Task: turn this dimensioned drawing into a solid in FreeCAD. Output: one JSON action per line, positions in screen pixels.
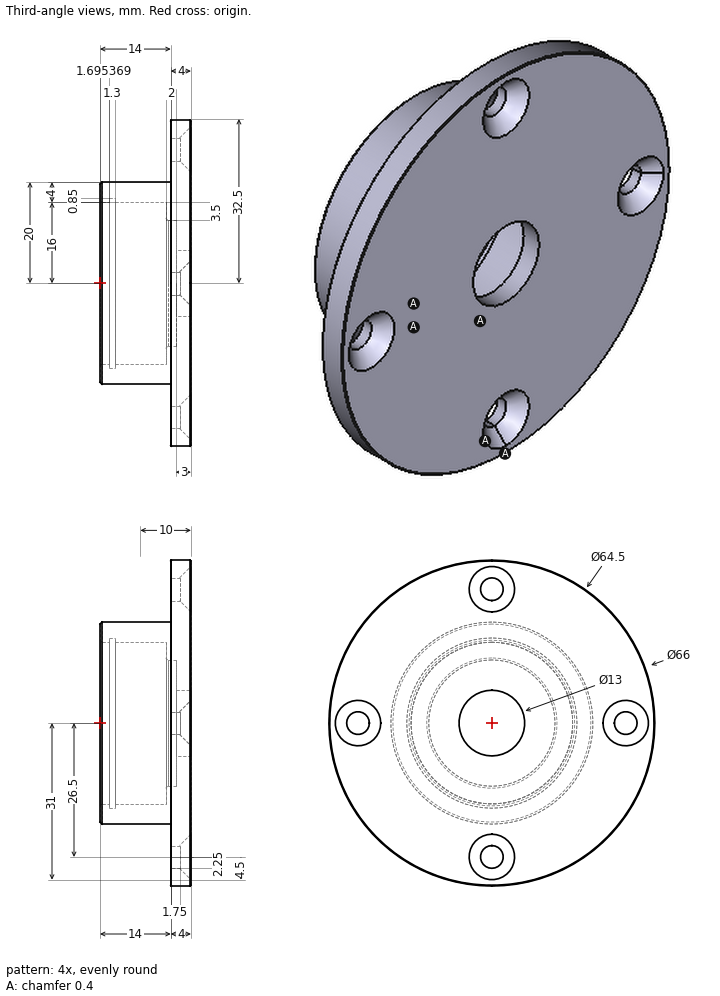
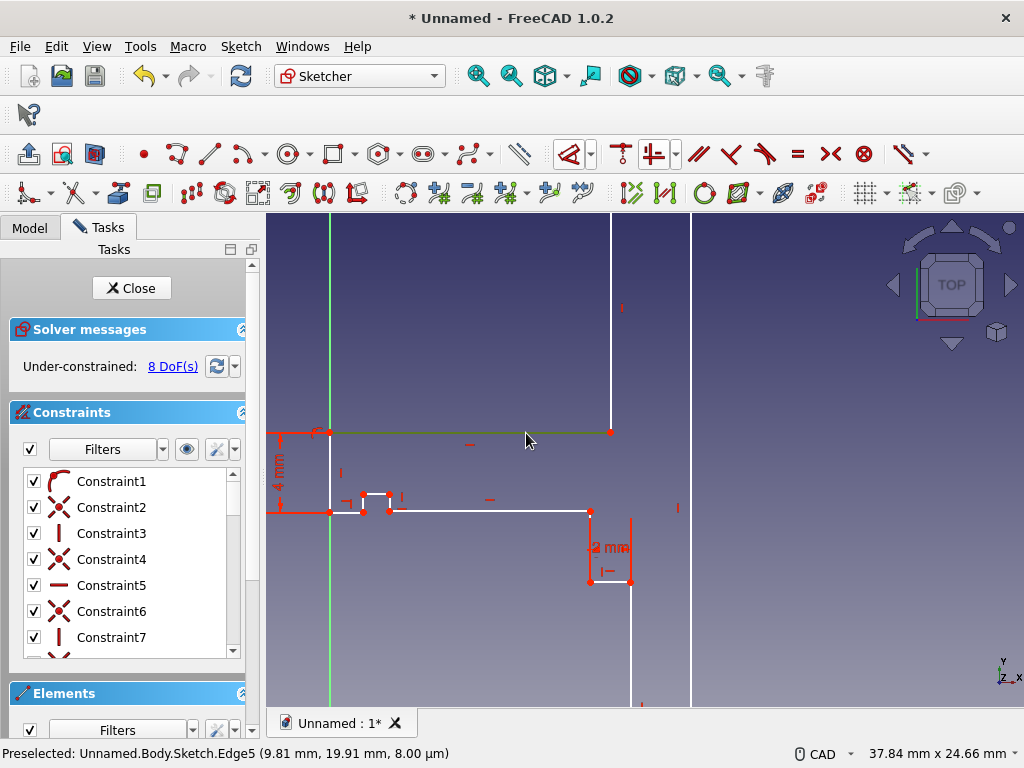
{"action": "left_click", "coordinate": [590, 154]}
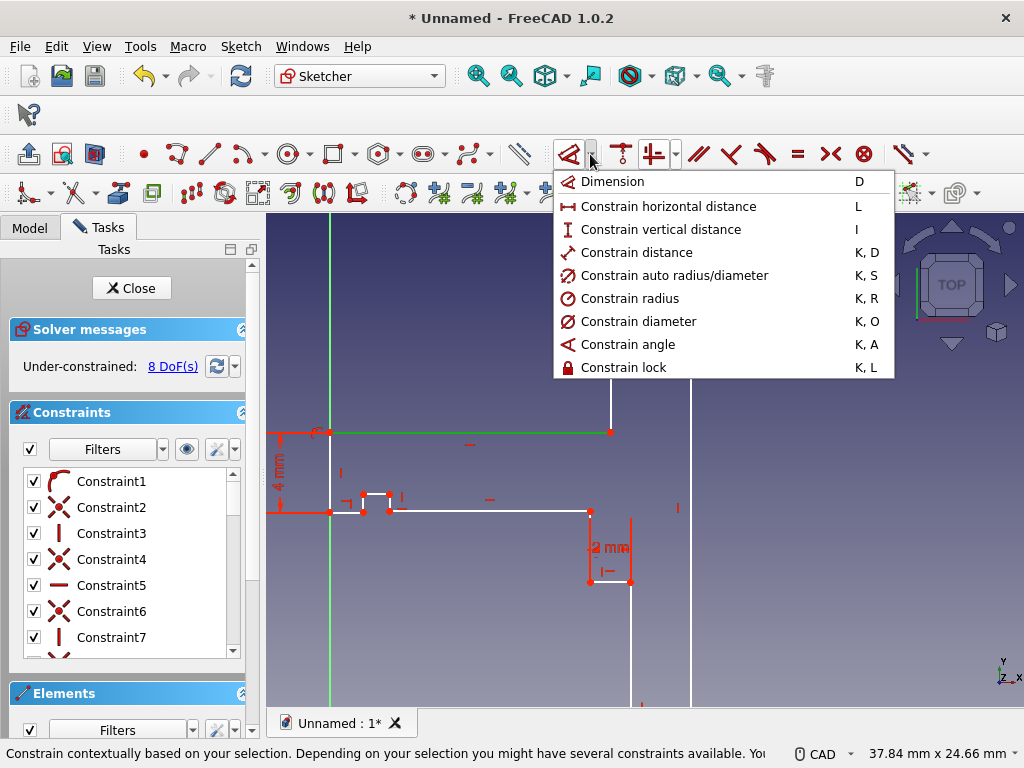
{"action": "left_click", "coordinate": [724, 206]}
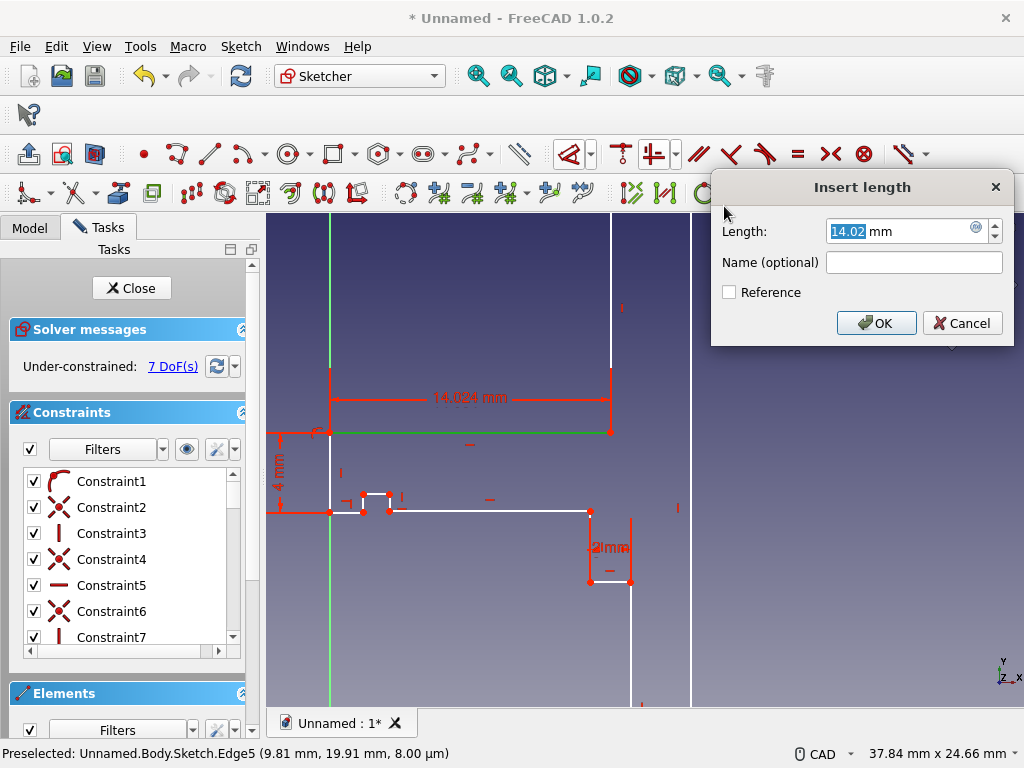
{"action": "type", "text": "14"}
{"action": "key", "text": "Return"}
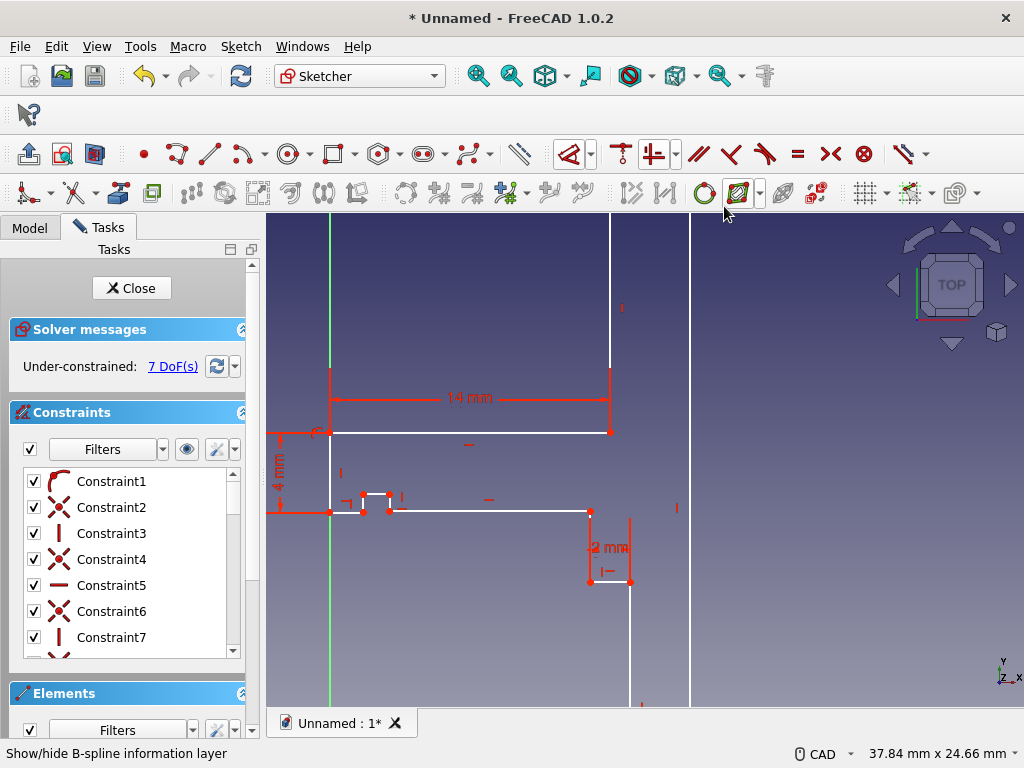
{"action": "scroll", "coordinate": [374, 494], "scroll_direction": "up", "scroll_amount": 3}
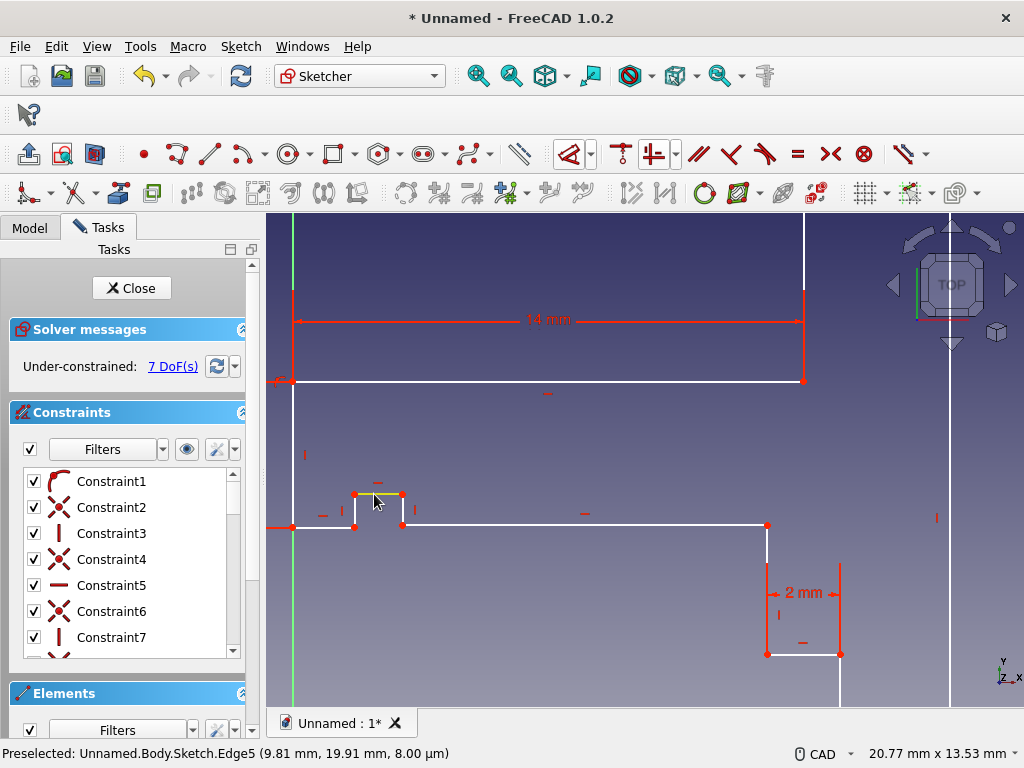
{"action": "left_click", "coordinate": [374, 494]}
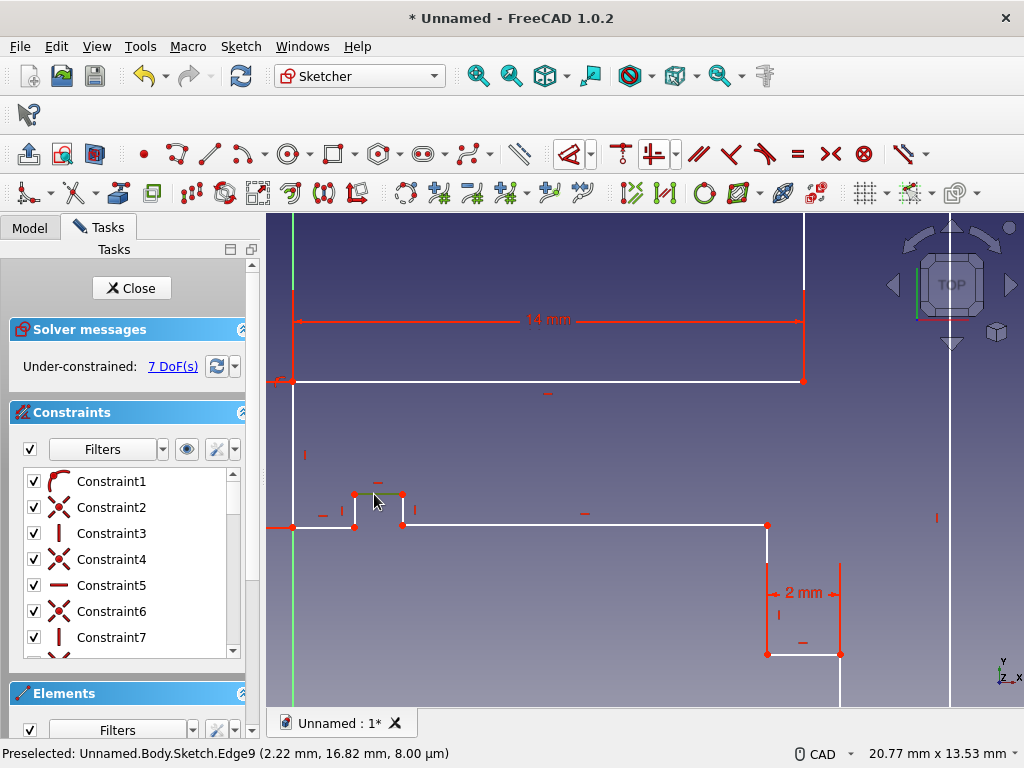
{"action": "key", "text": "l"}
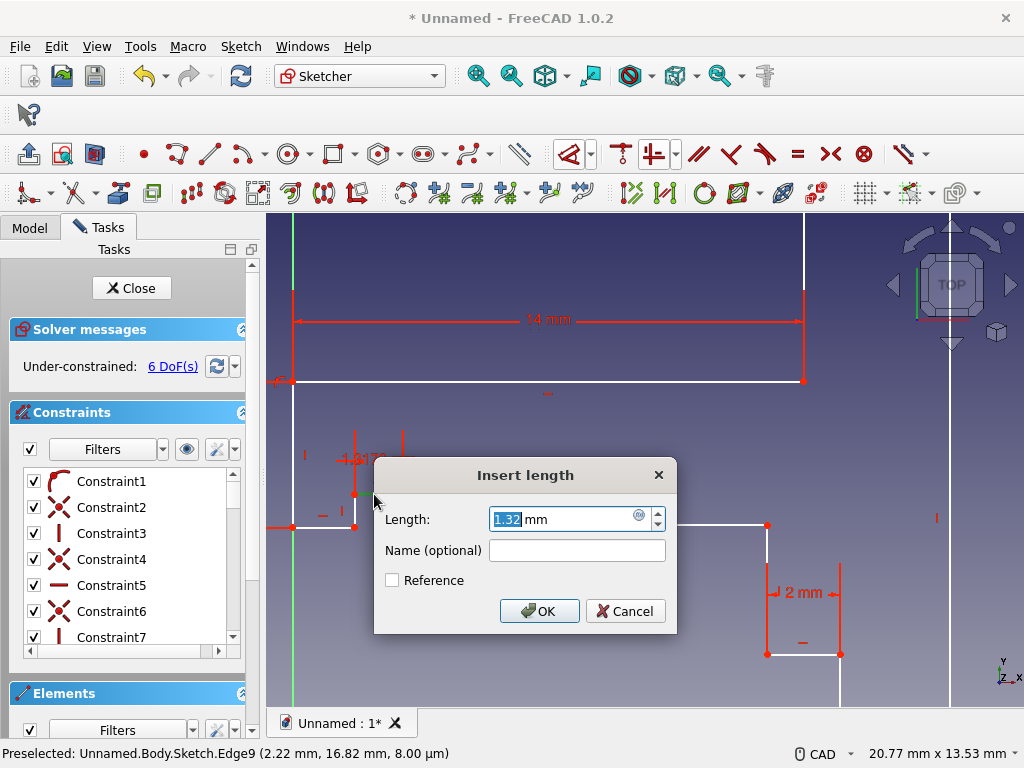
{"action": "type", "text": "1.3"}
{"action": "key", "text": "Return"}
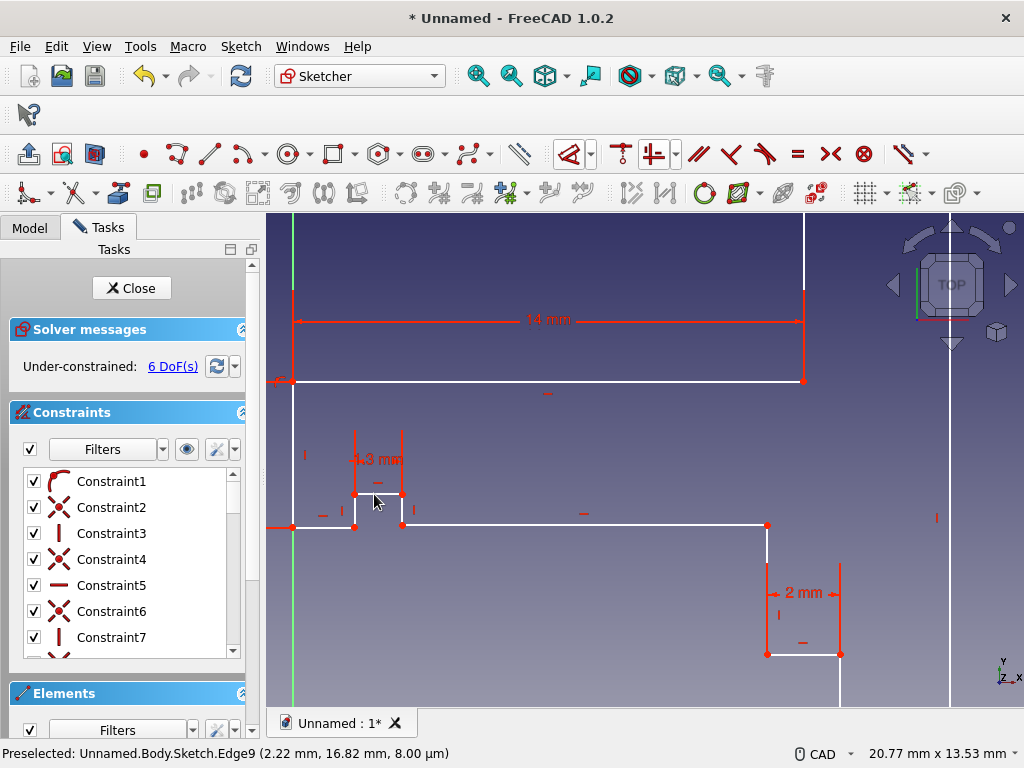
{"action": "left_click", "coordinate": [767, 564]}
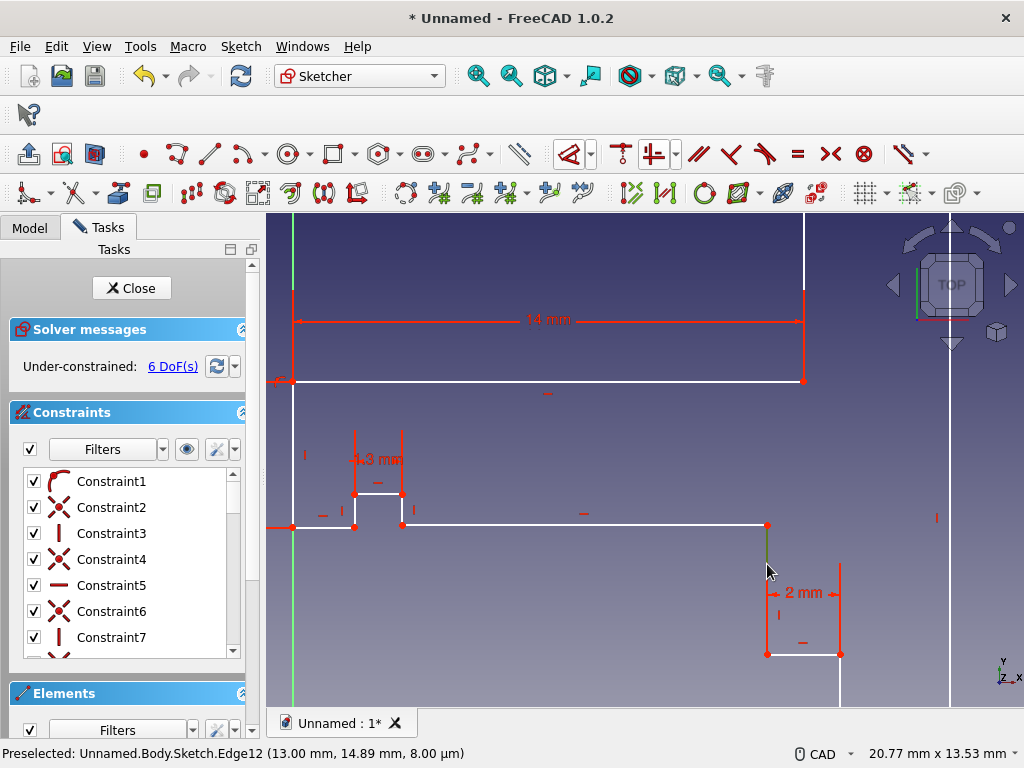
{"action": "left_click", "coordinate": [590, 154]}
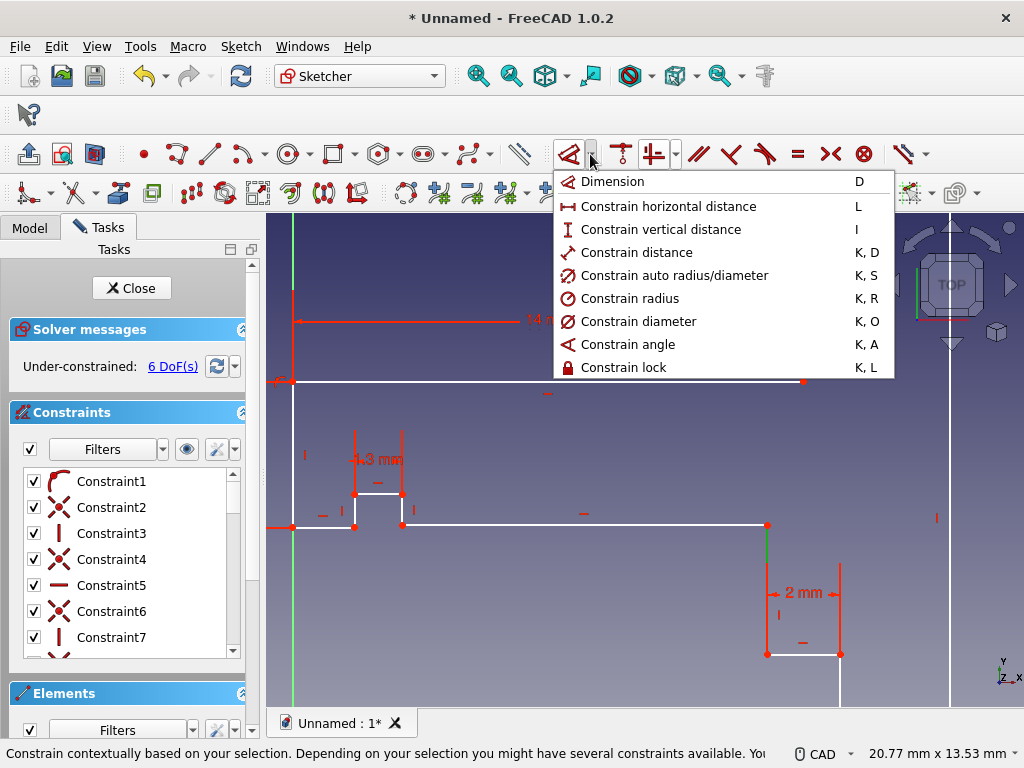
{"action": "left_click", "coordinate": [724, 230]}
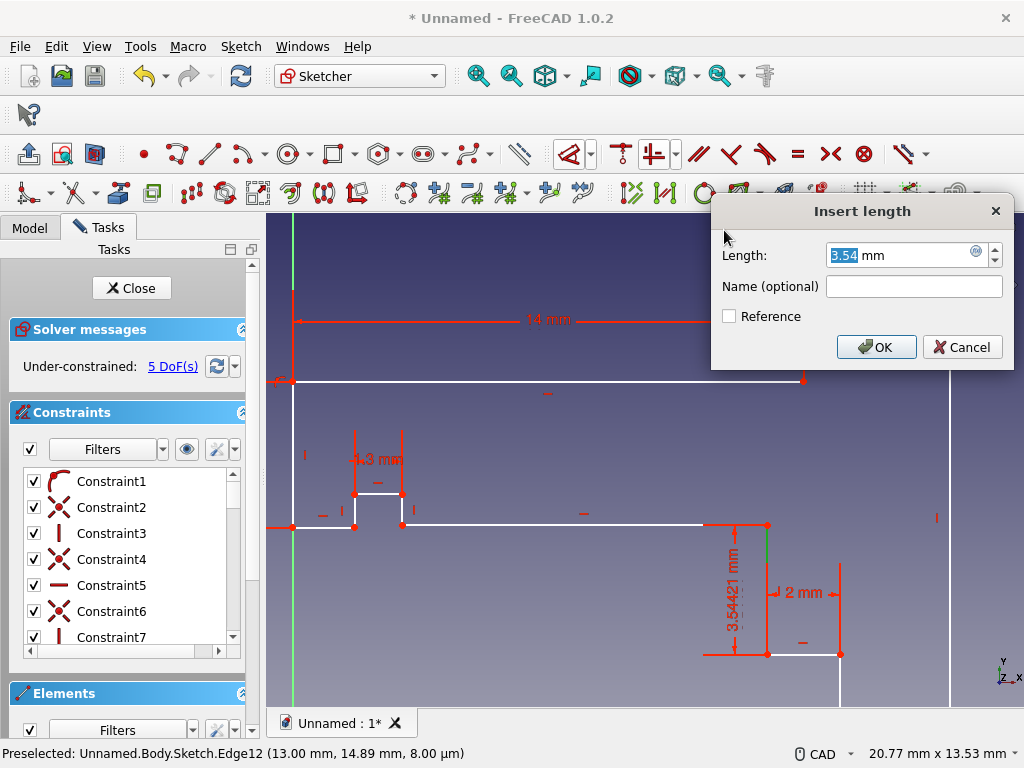
{"action": "type", "text": "3.5"}
{"action": "key", "text": "Return"}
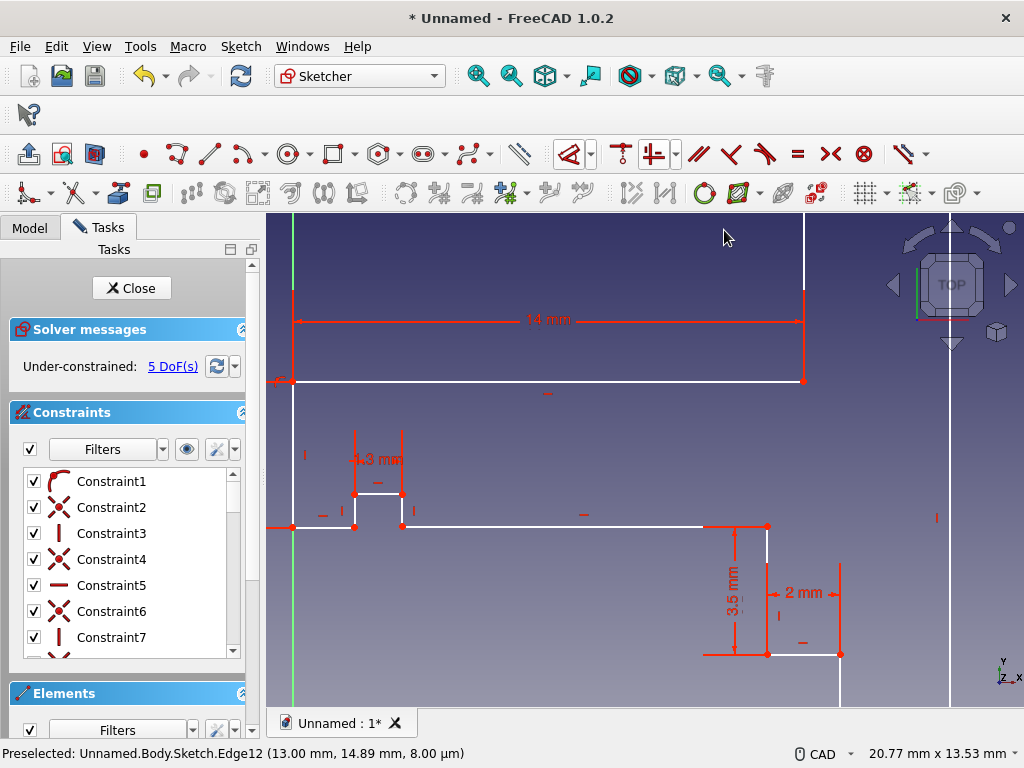
{"action": "scroll", "coordinate": [562, 442], "scroll_direction": "down", "scroll_amount": 7}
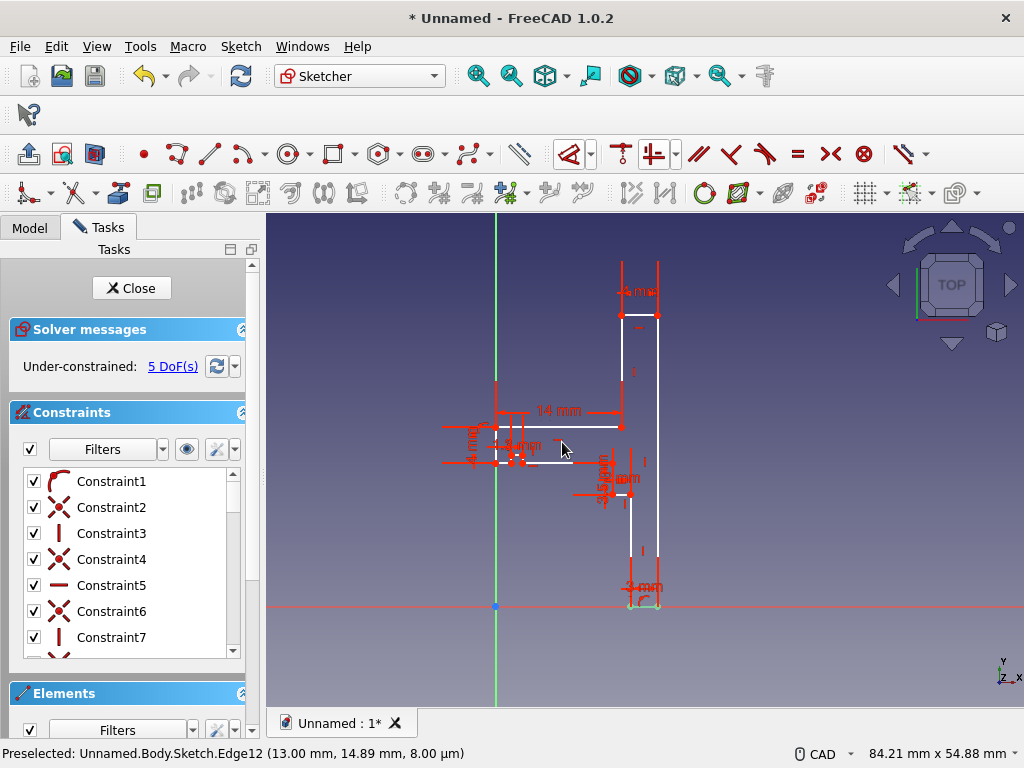
{"action": "left_click", "coordinate": [622, 427]}